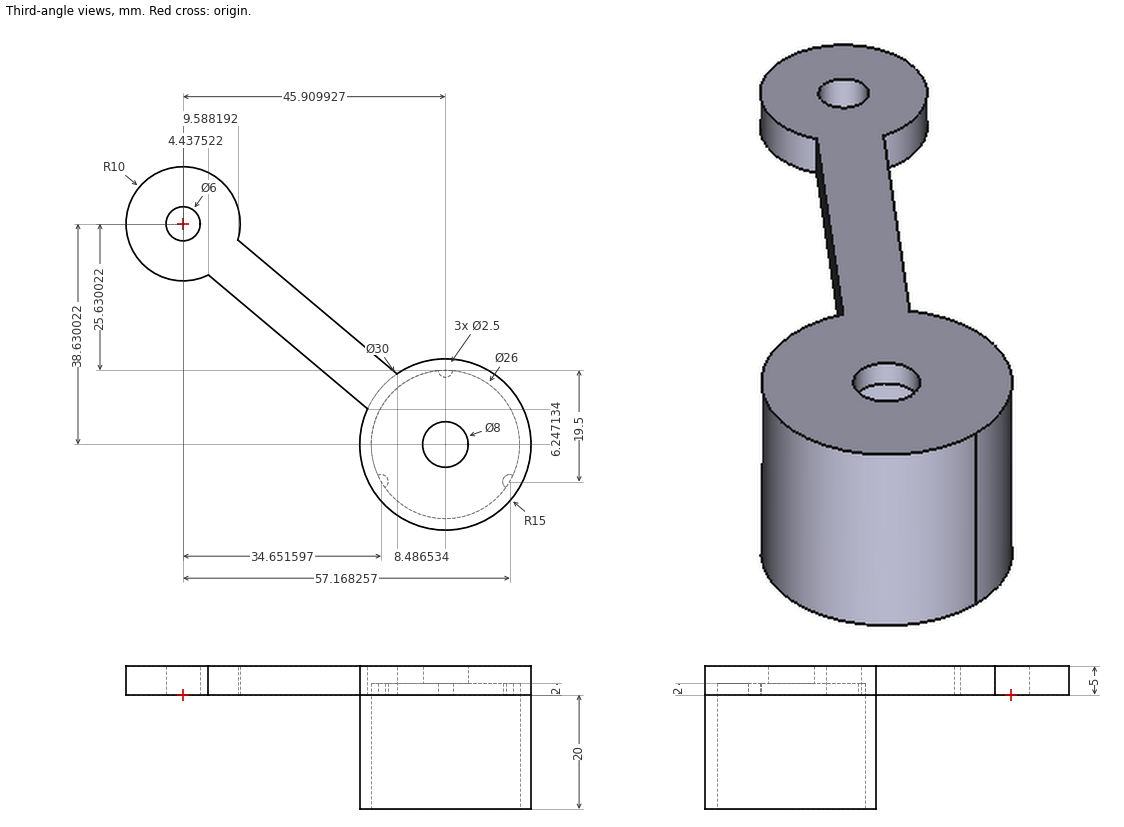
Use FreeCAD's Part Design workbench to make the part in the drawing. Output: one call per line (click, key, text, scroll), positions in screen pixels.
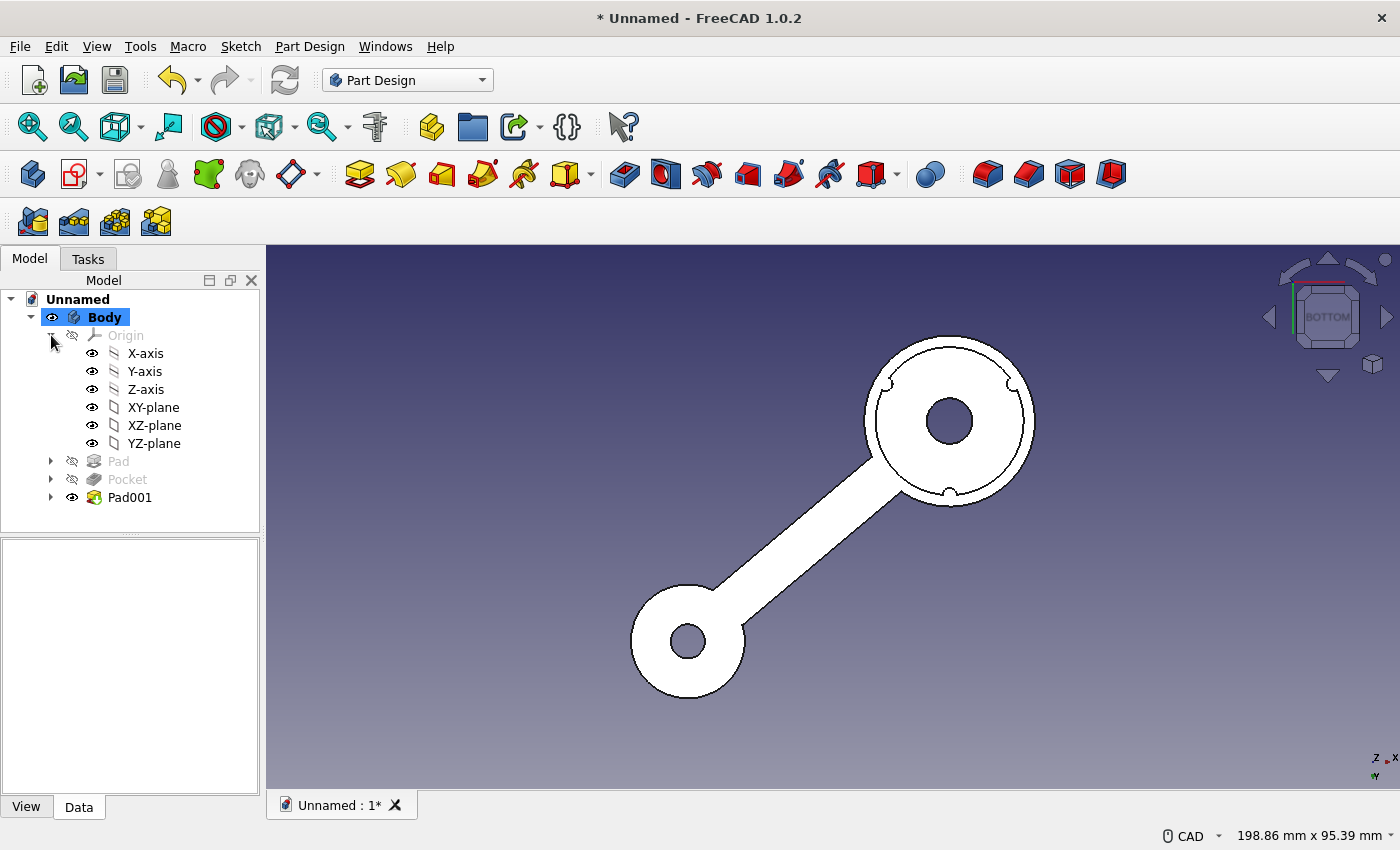
click(137, 407)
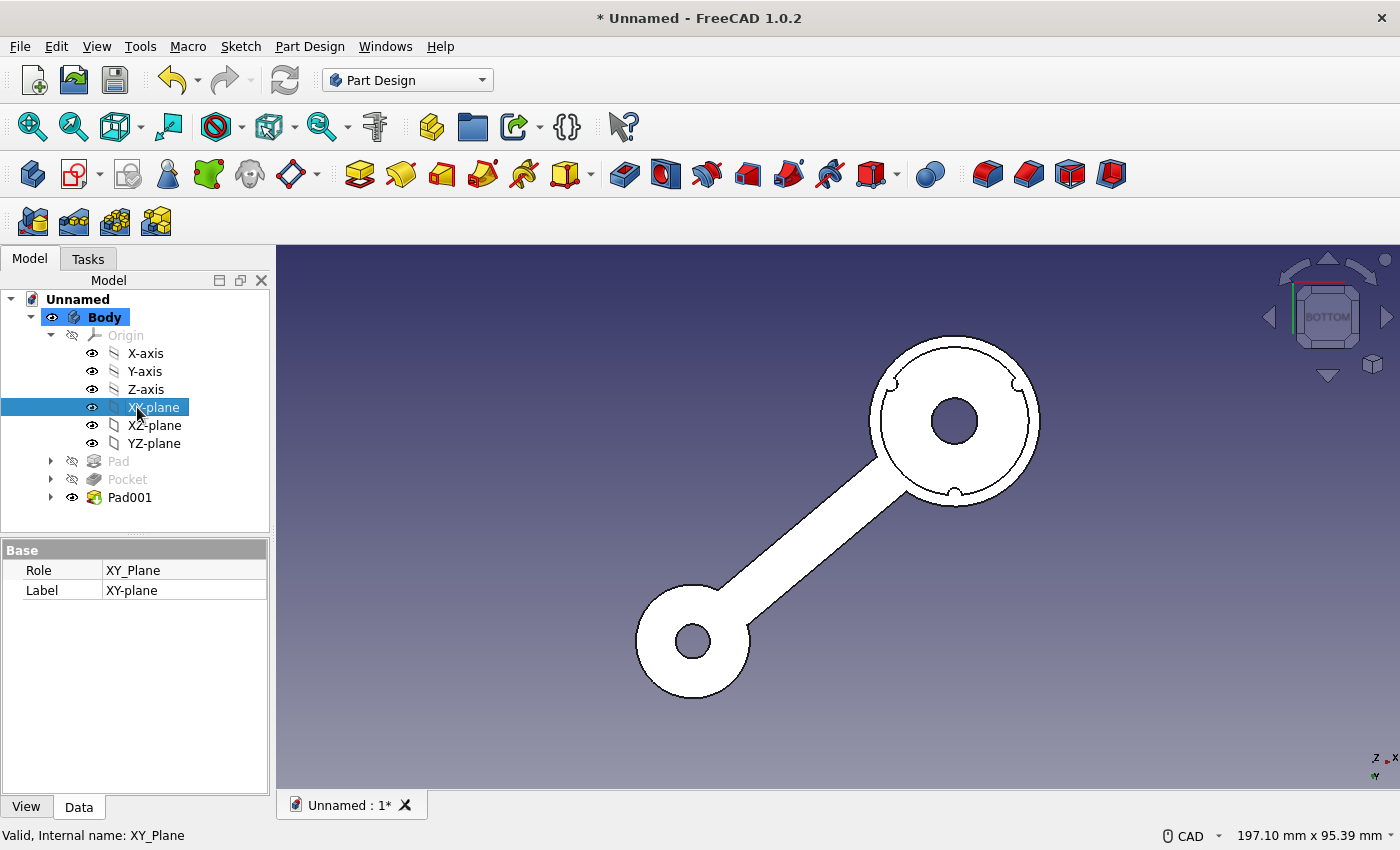
click(290, 174)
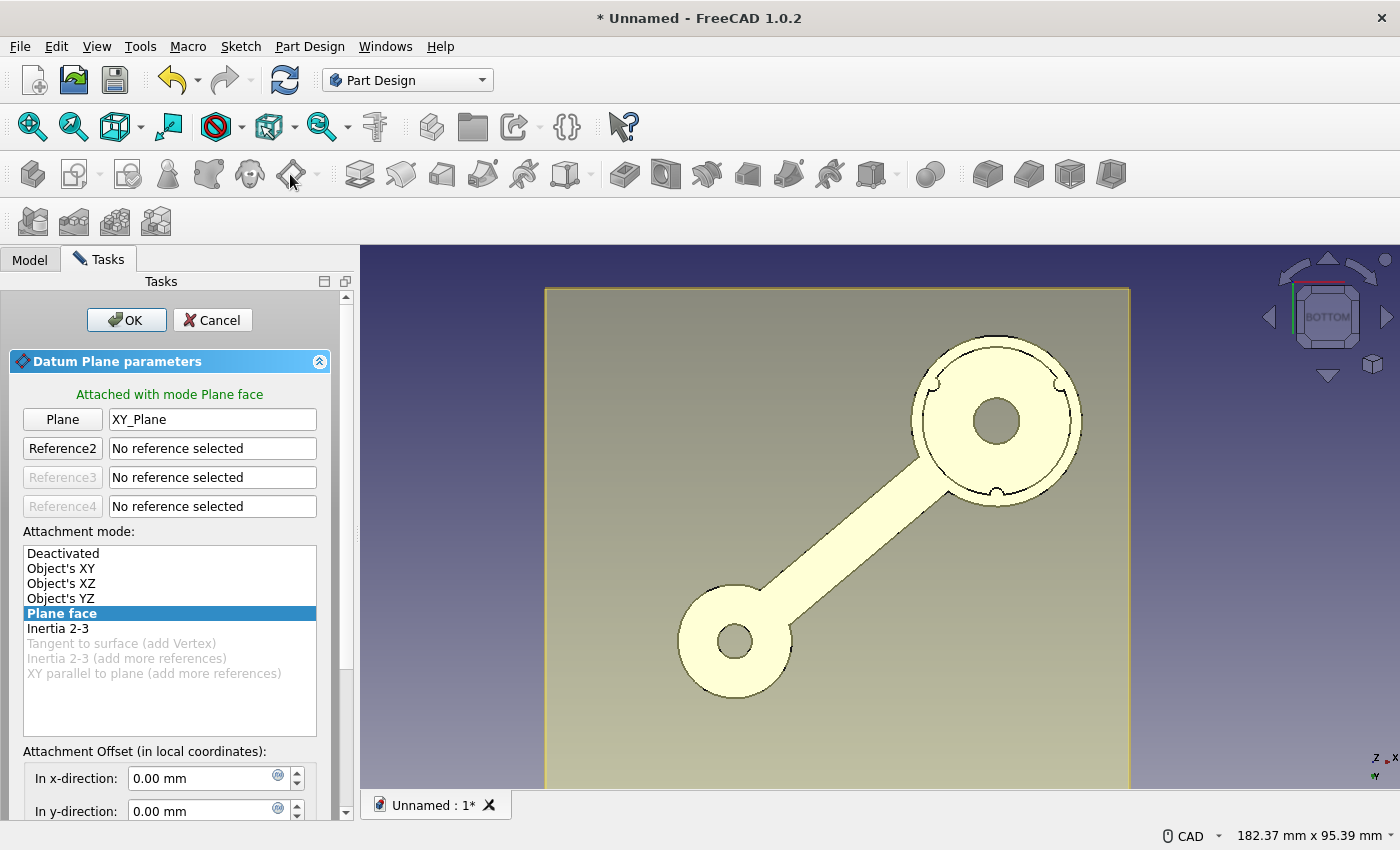
scroll(346, 556, down, 2)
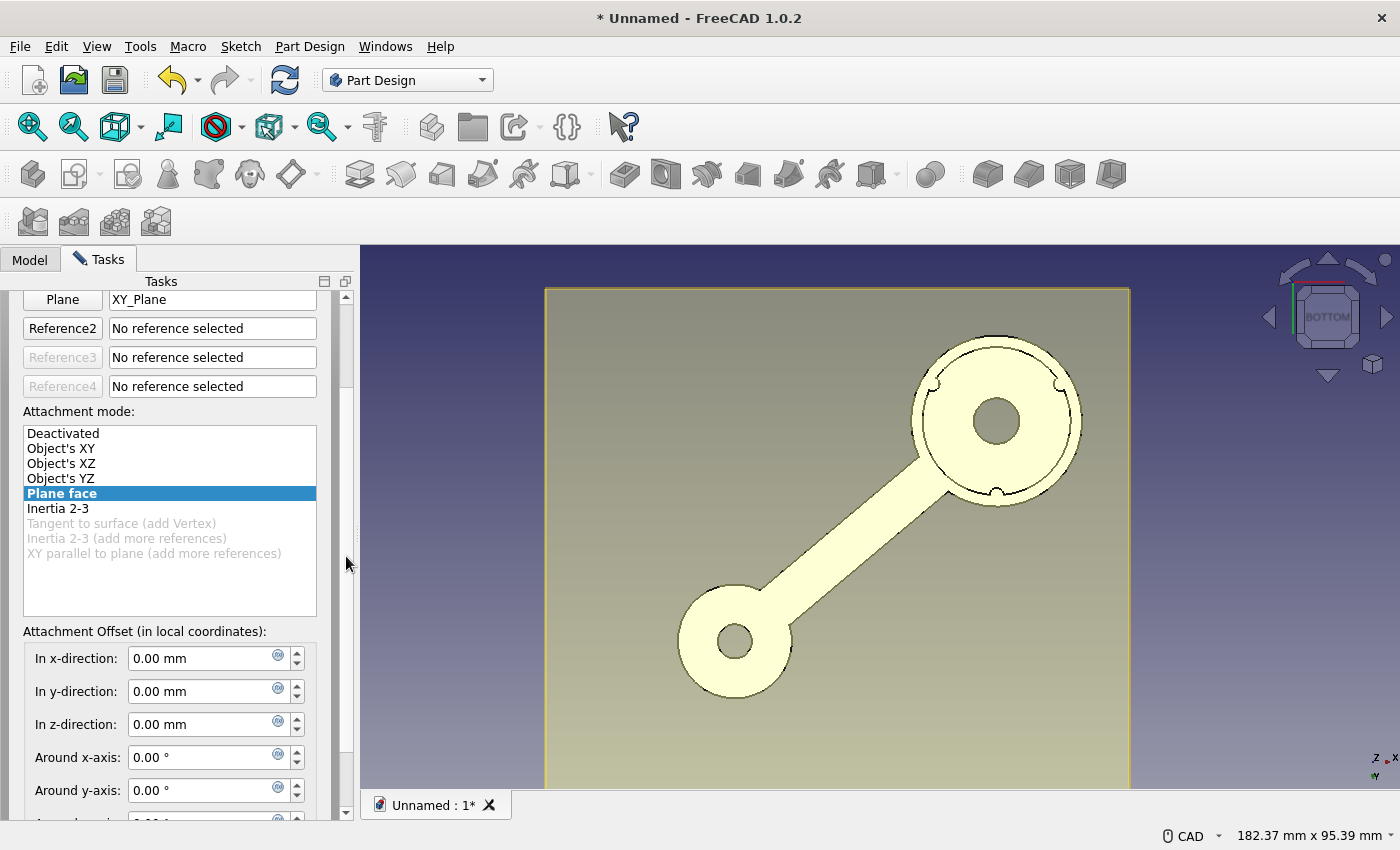
triple_click(210, 724)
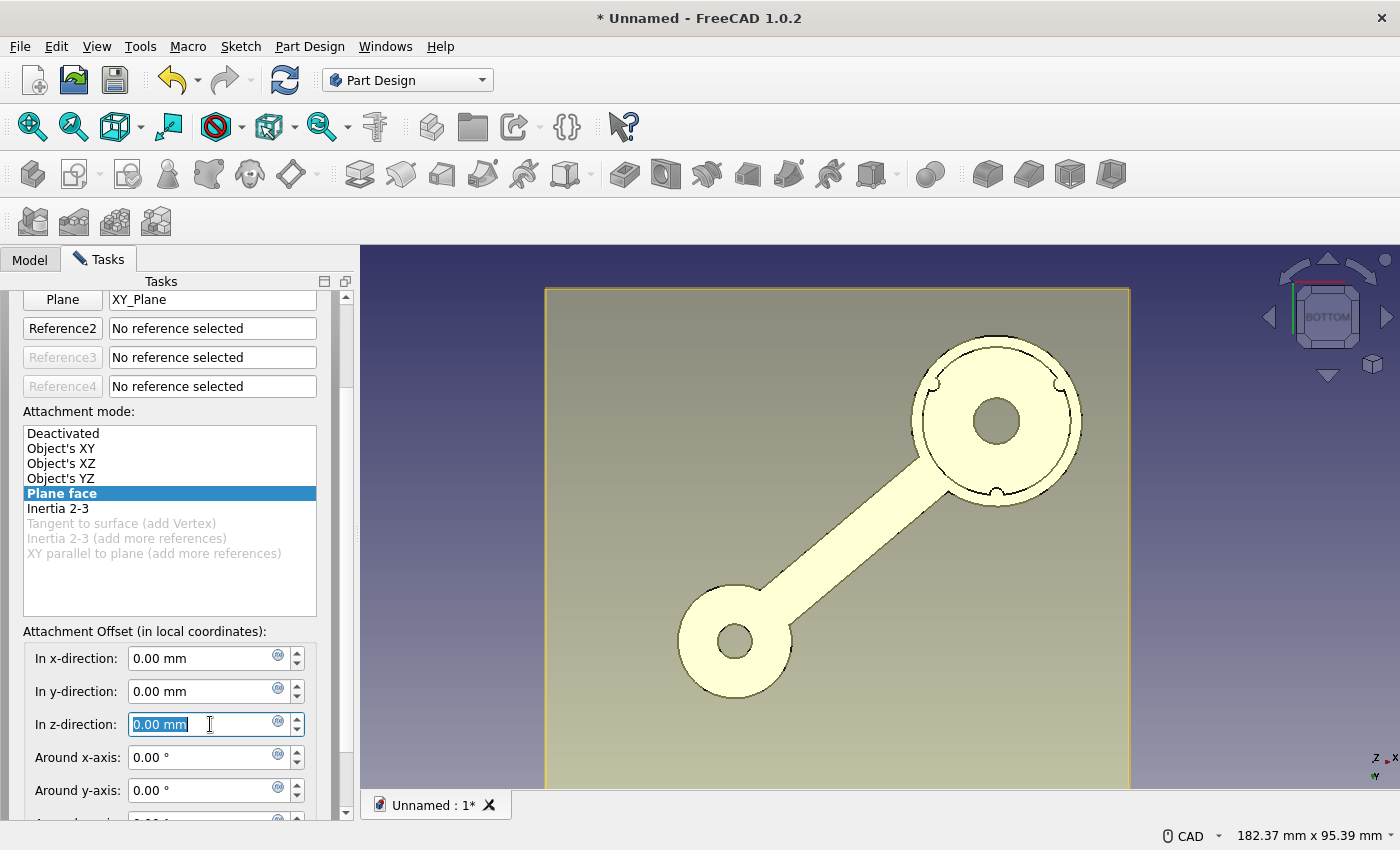
text(-20)
key(Tab)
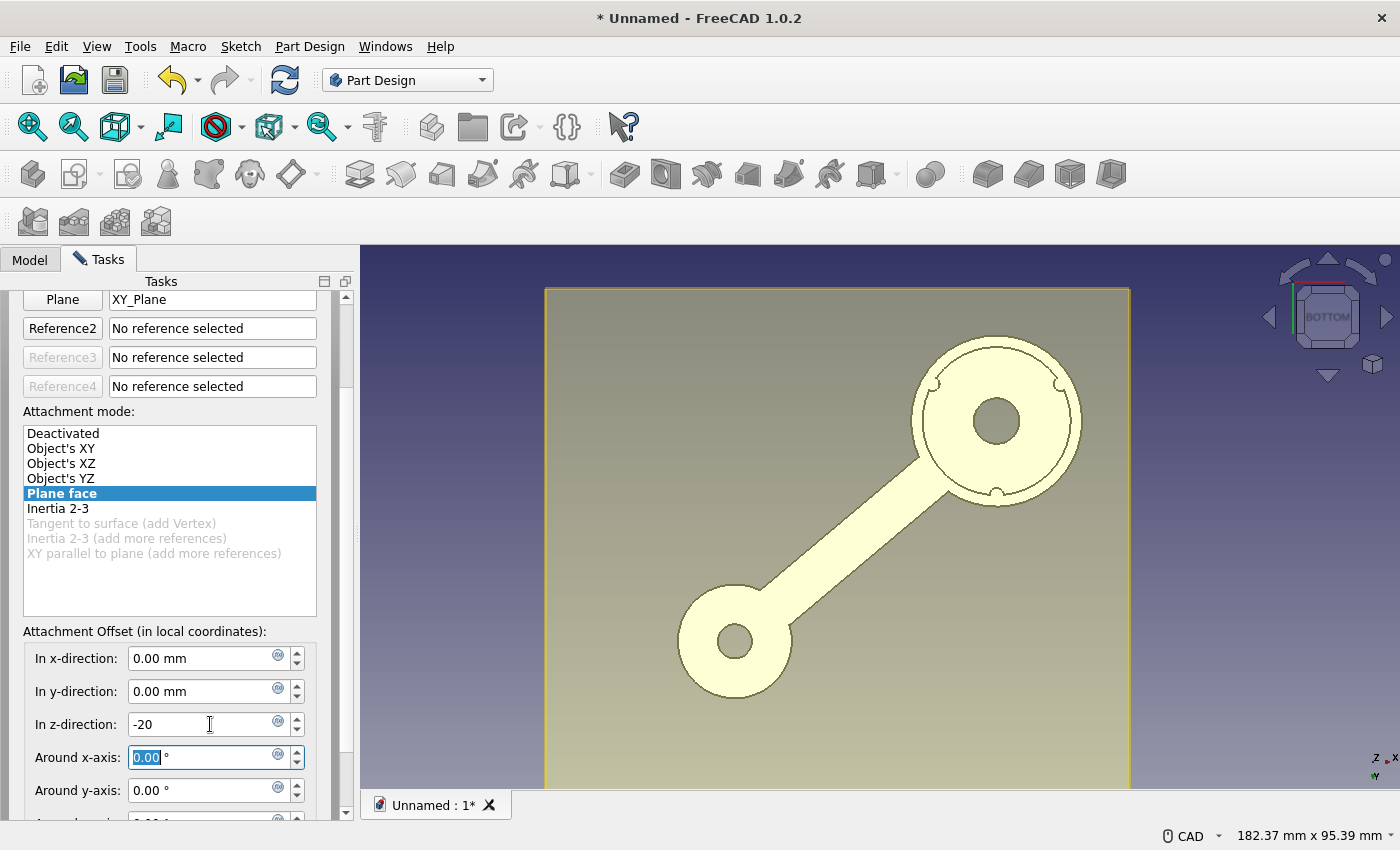
scroll(346, 556, up, 3)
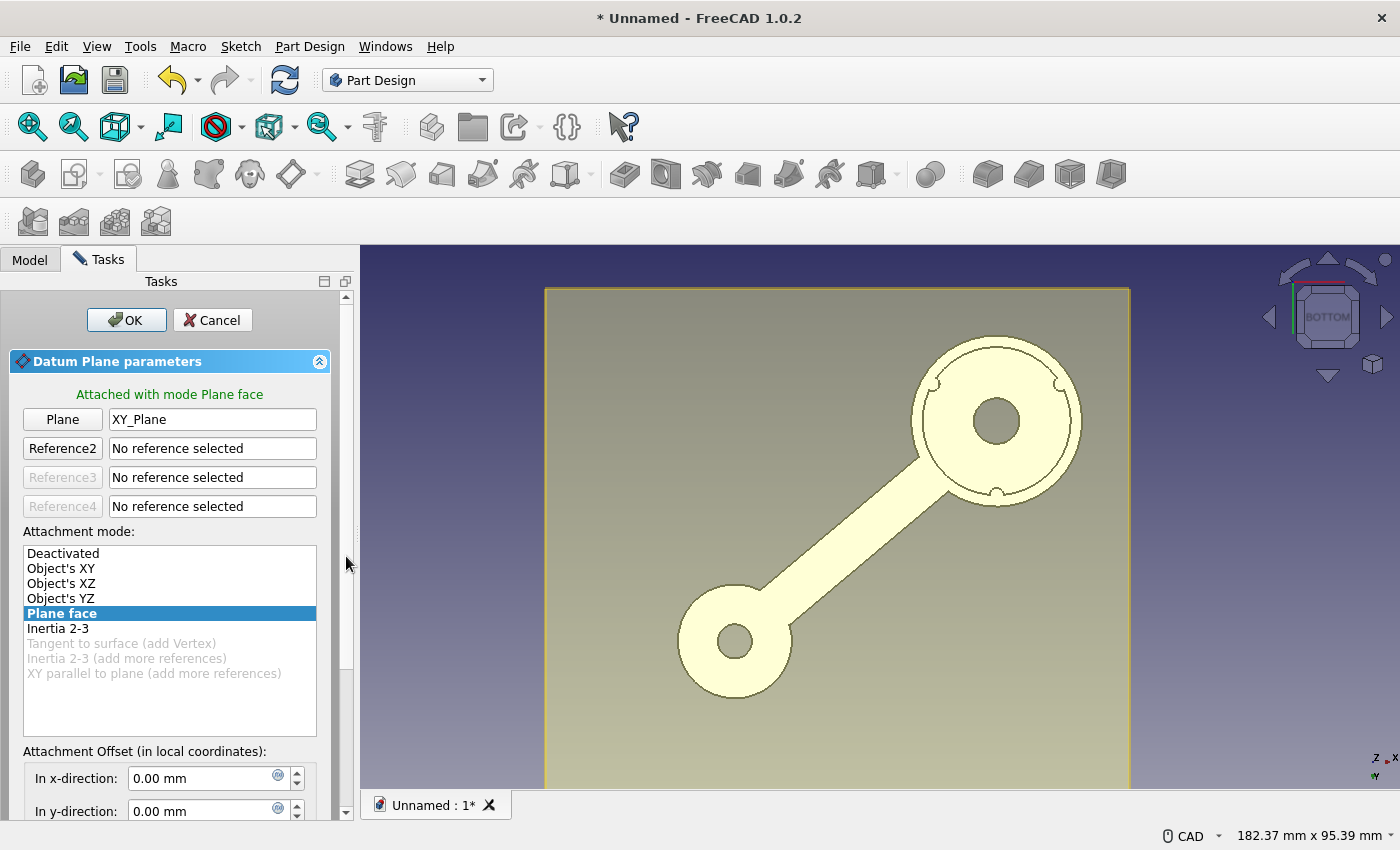
click(127, 320)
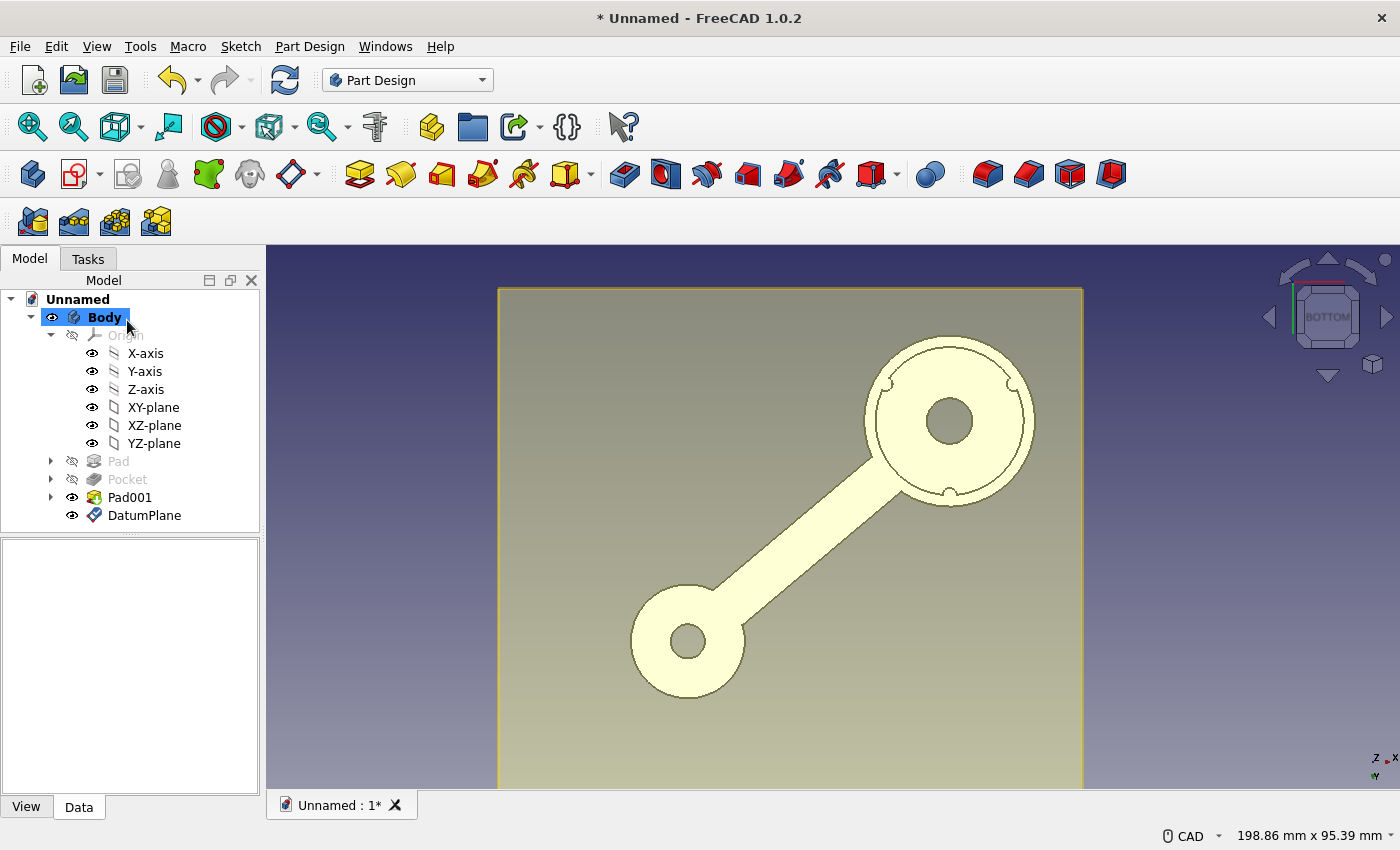
click(117, 515)